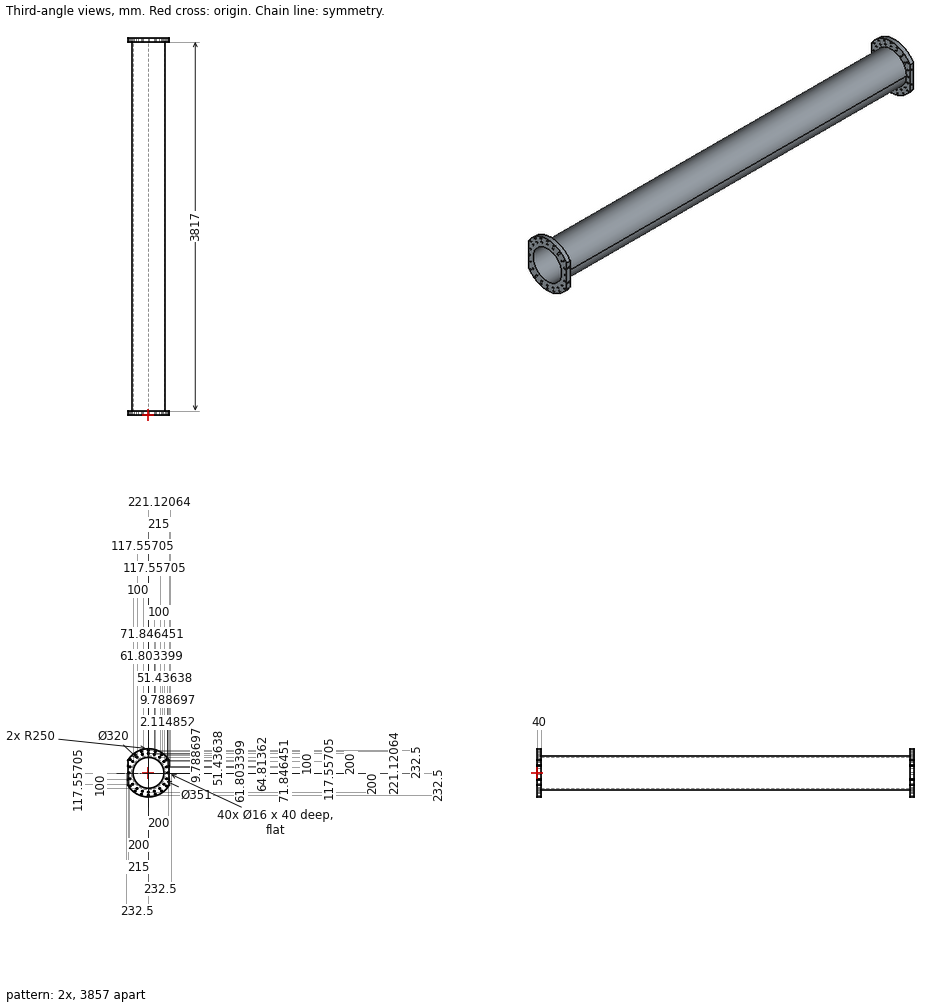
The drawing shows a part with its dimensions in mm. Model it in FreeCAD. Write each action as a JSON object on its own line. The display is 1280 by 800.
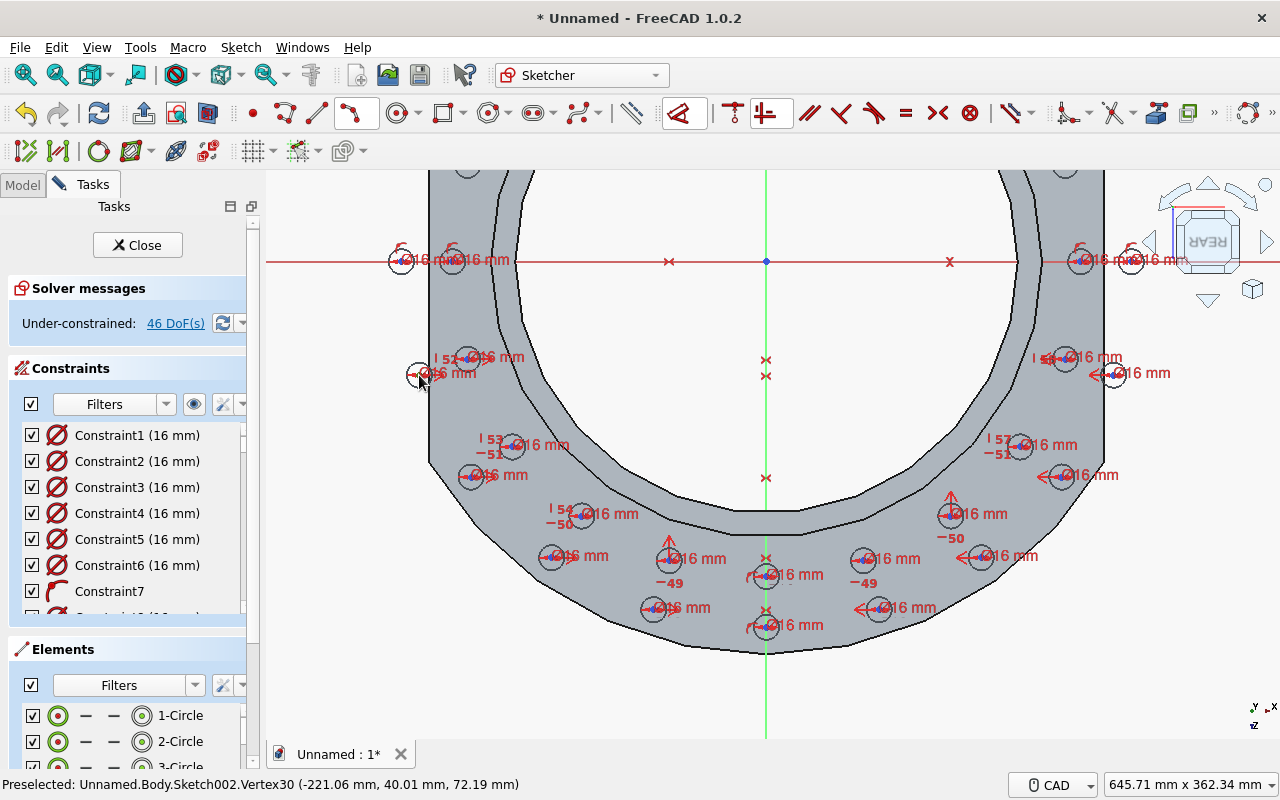
{"action": "scroll", "coordinate": [654, 612], "scroll_direction": "down", "scroll_amount": 4}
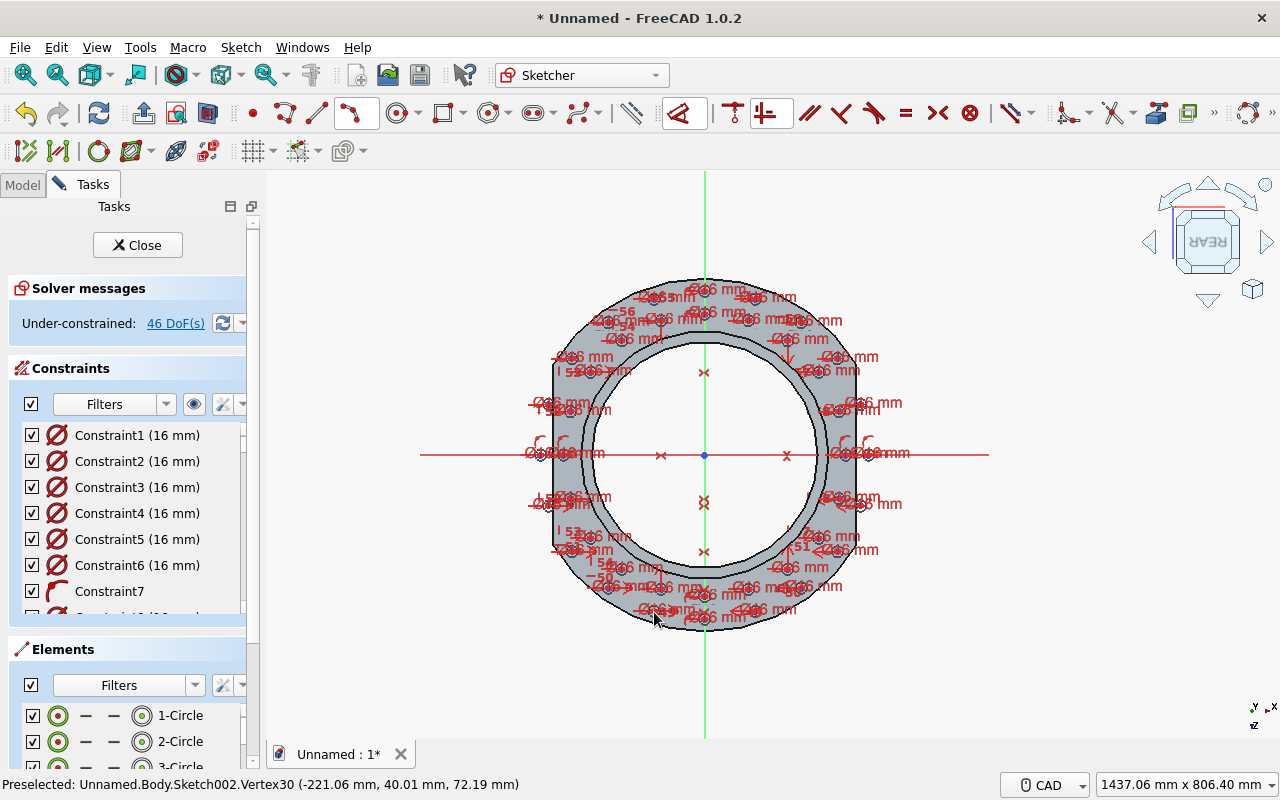
{"action": "left_click", "coordinate": [547, 403]}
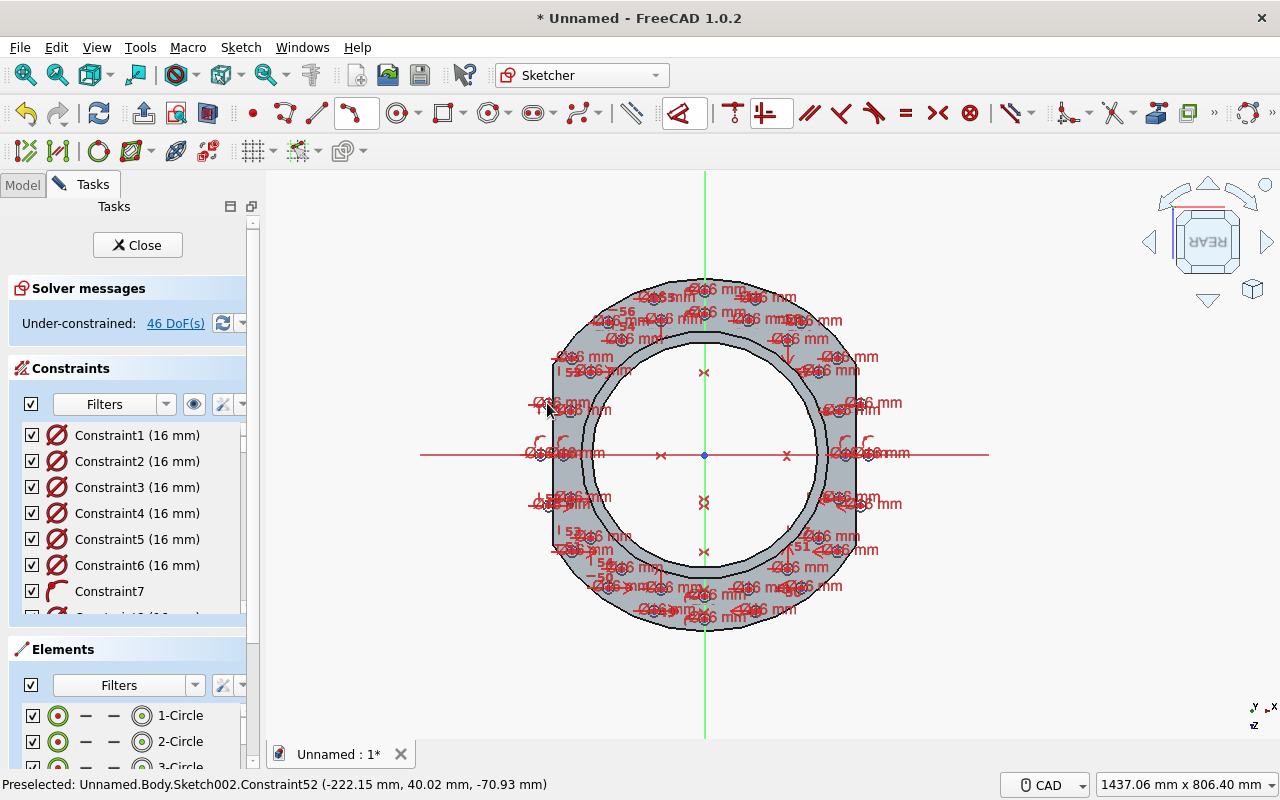
{"action": "left_click", "coordinate": [470, 455]}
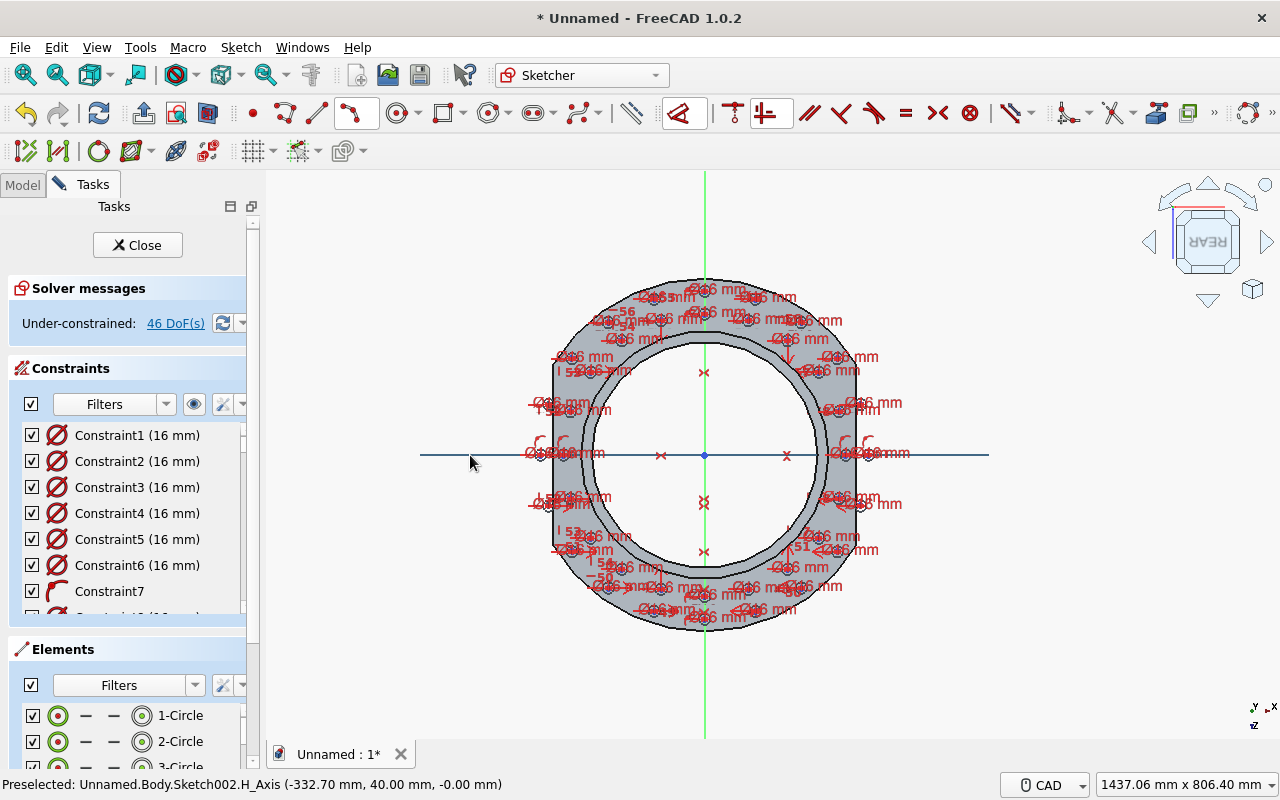
{"action": "left_click", "coordinate": [938, 114]}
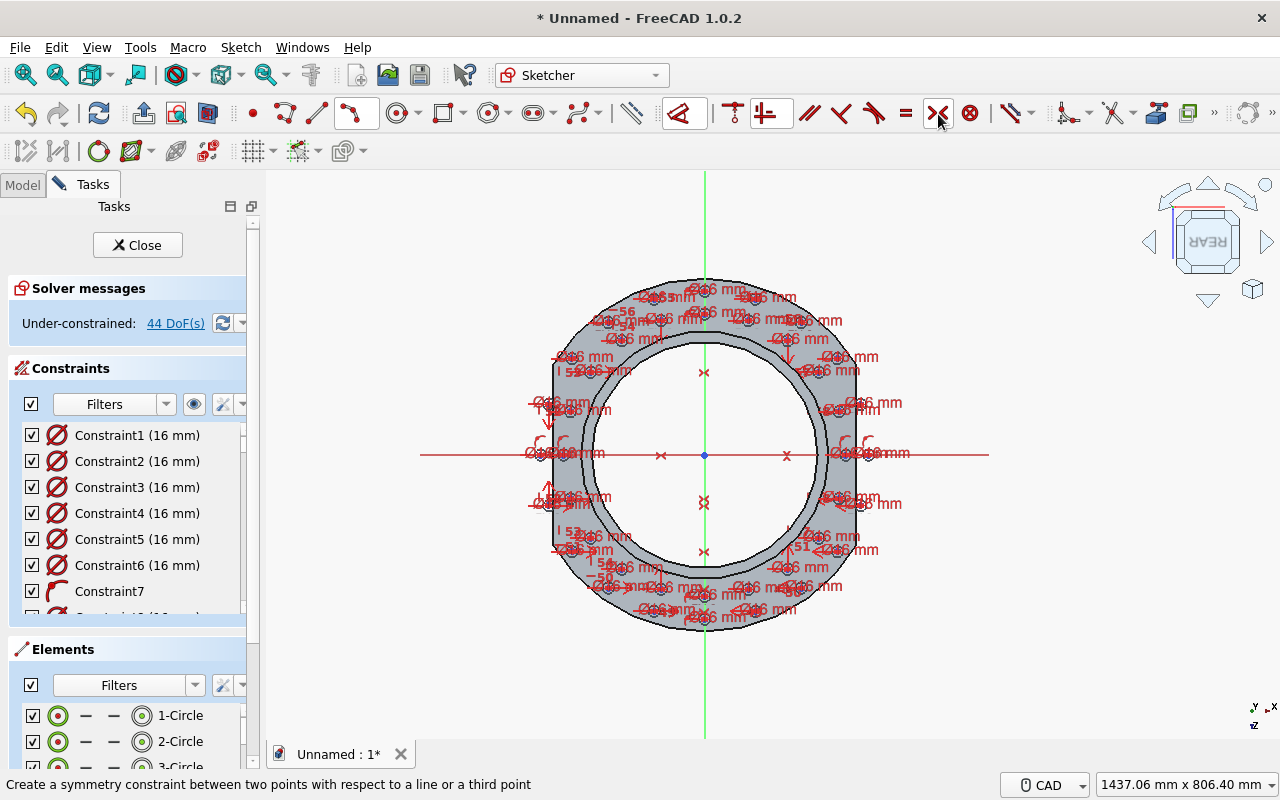
{"action": "left_click", "coordinate": [572, 552]}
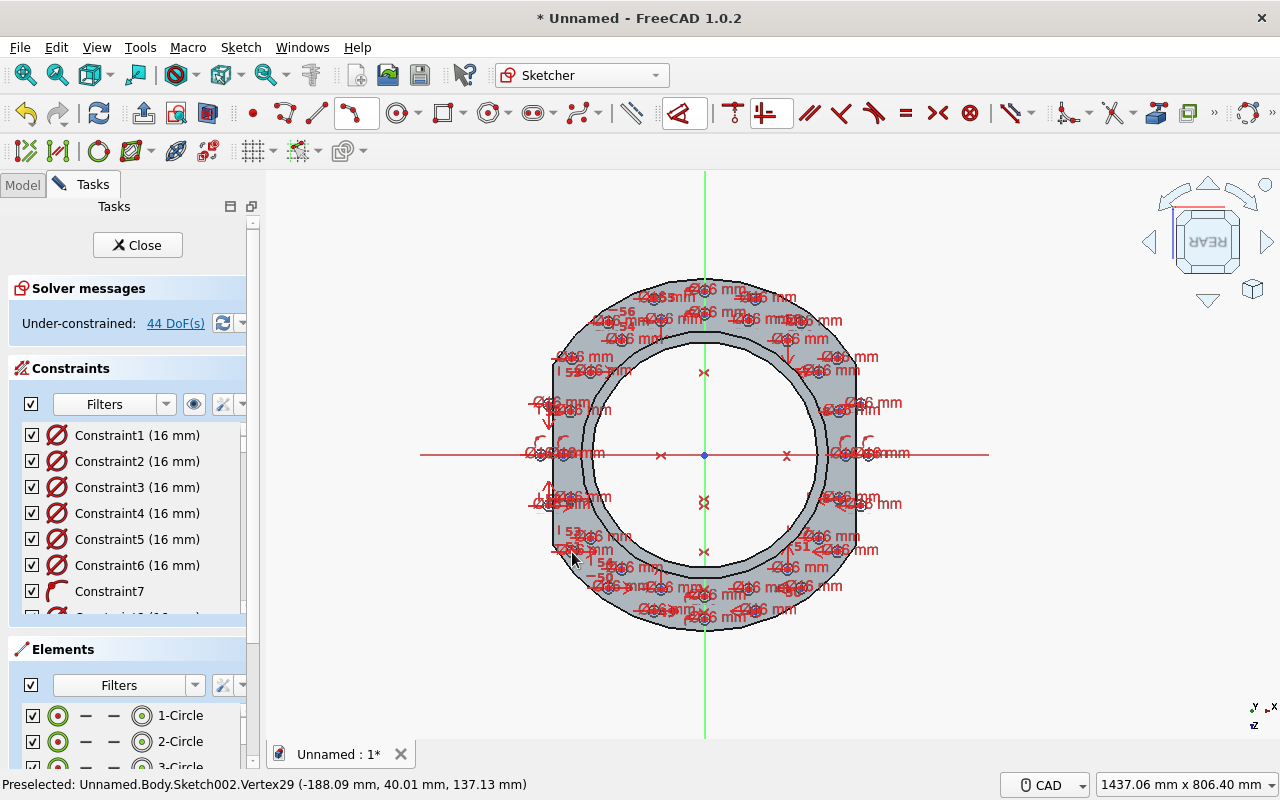
{"action": "left_click", "coordinate": [572, 359]}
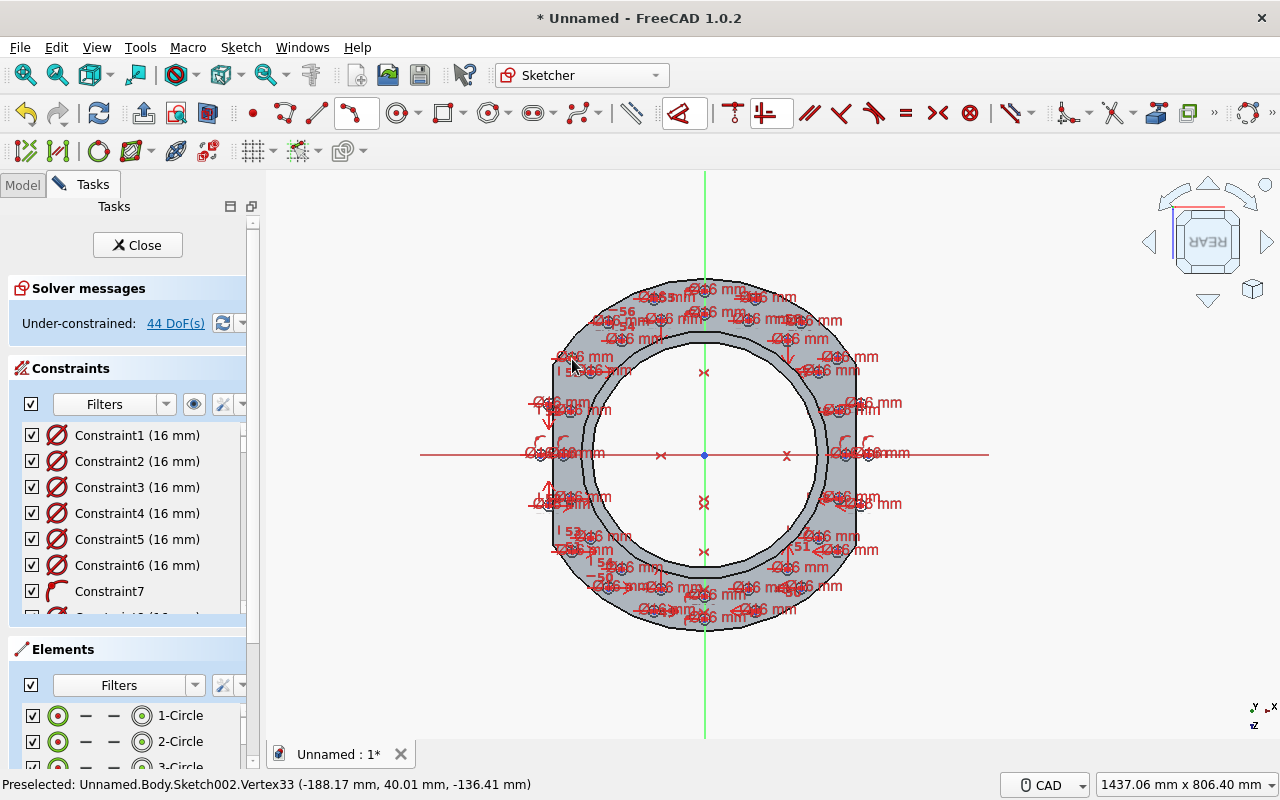
{"action": "left_click", "coordinate": [470, 455]}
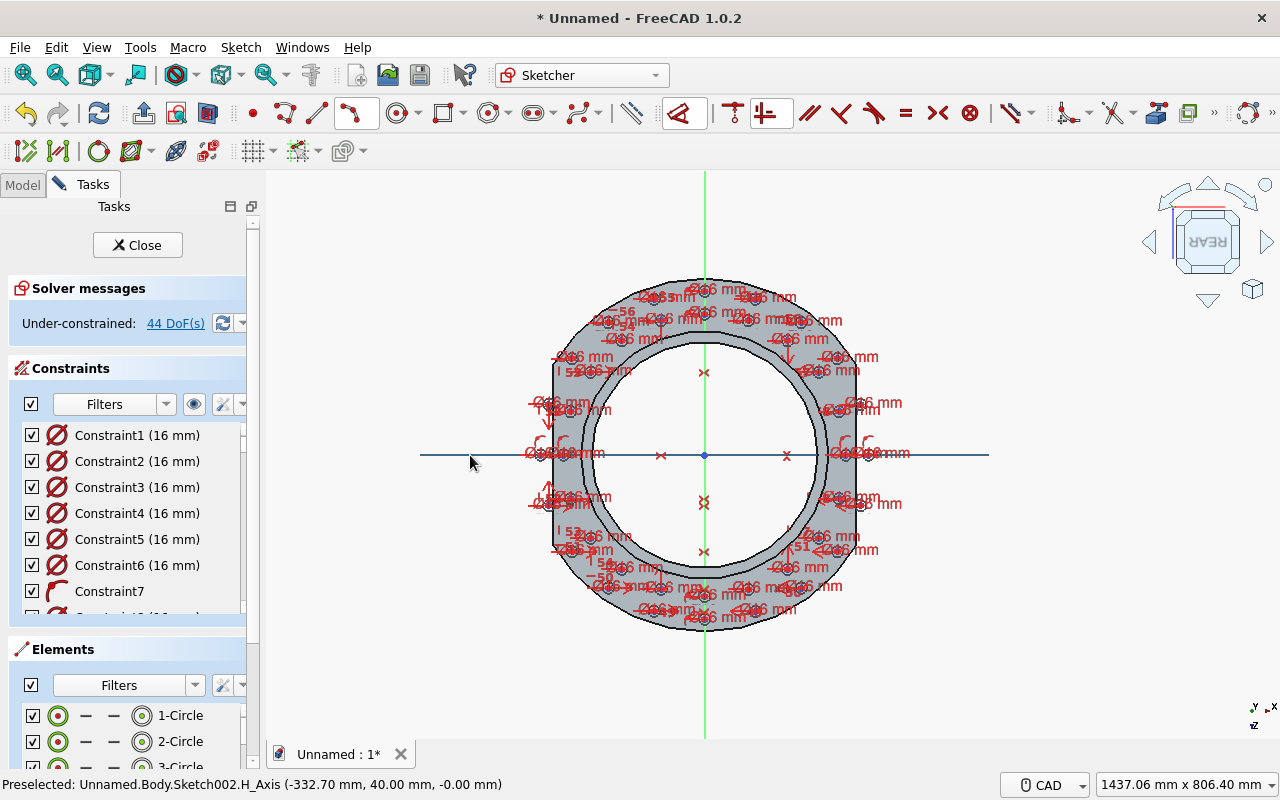
{"action": "left_click", "coordinate": [938, 114]}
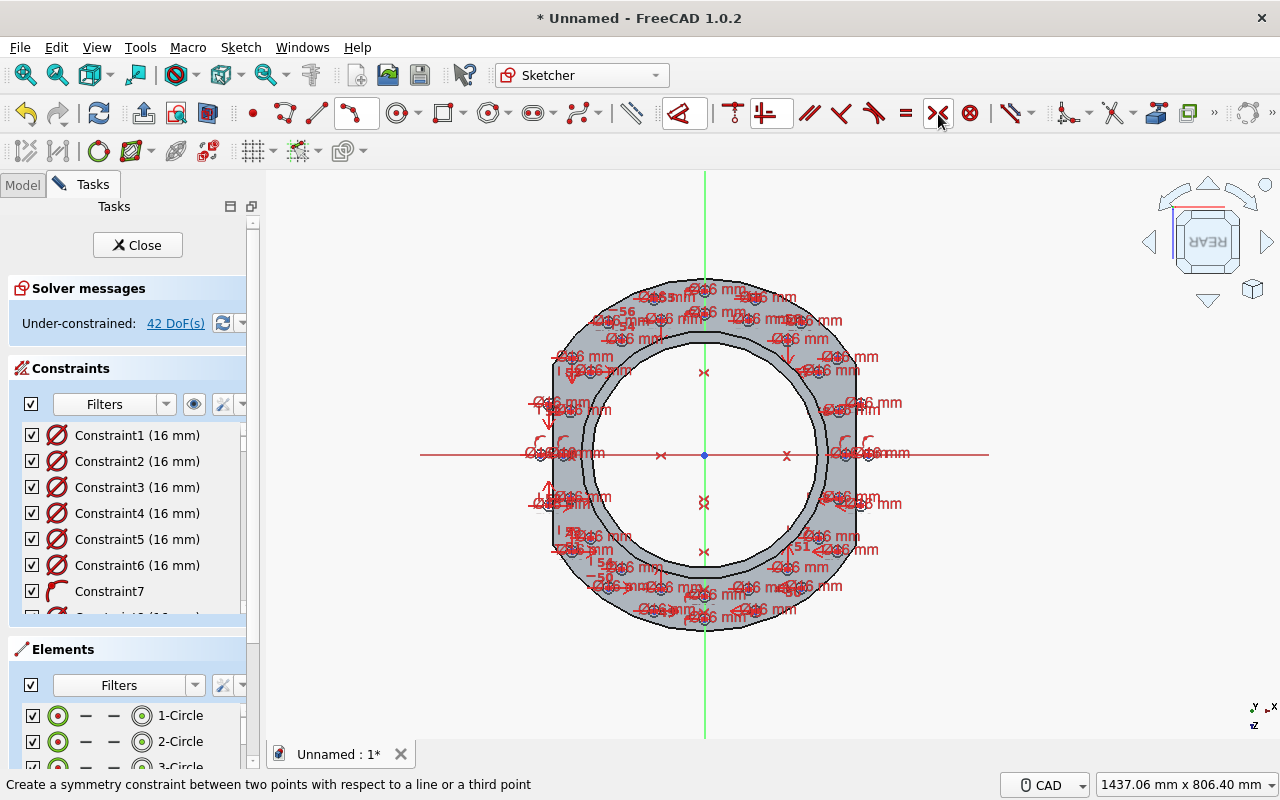
{"action": "left_click", "coordinate": [608, 588]}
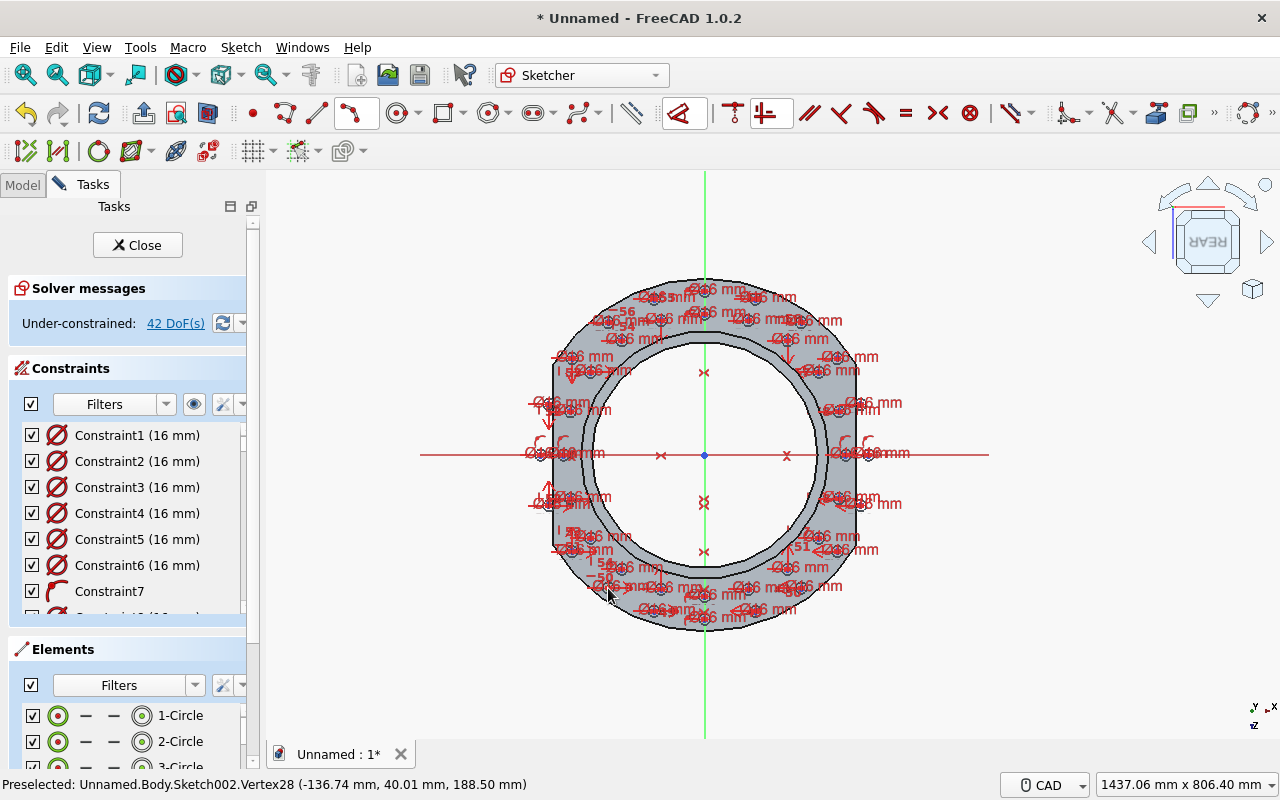
{"action": "left_click", "coordinate": [608, 323]}